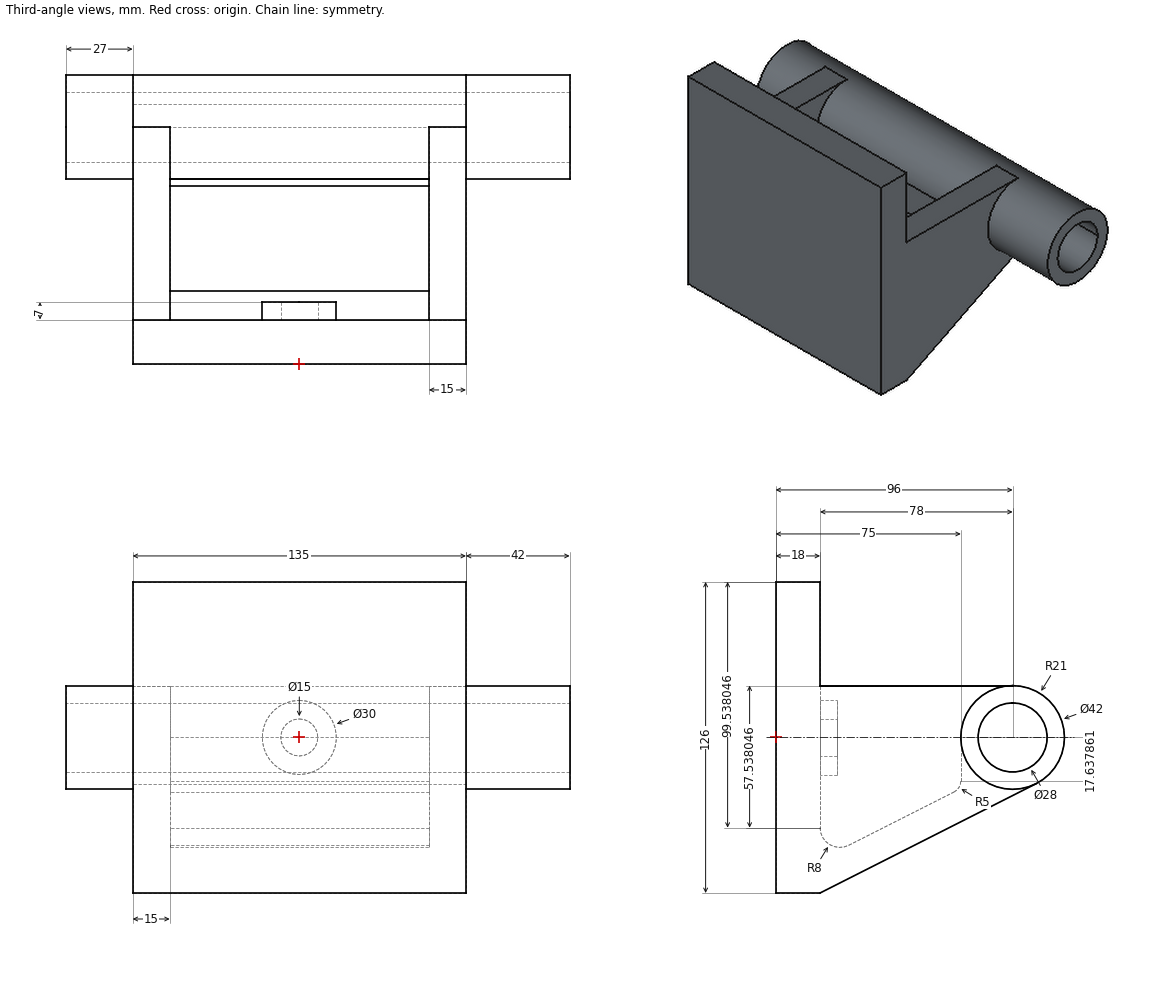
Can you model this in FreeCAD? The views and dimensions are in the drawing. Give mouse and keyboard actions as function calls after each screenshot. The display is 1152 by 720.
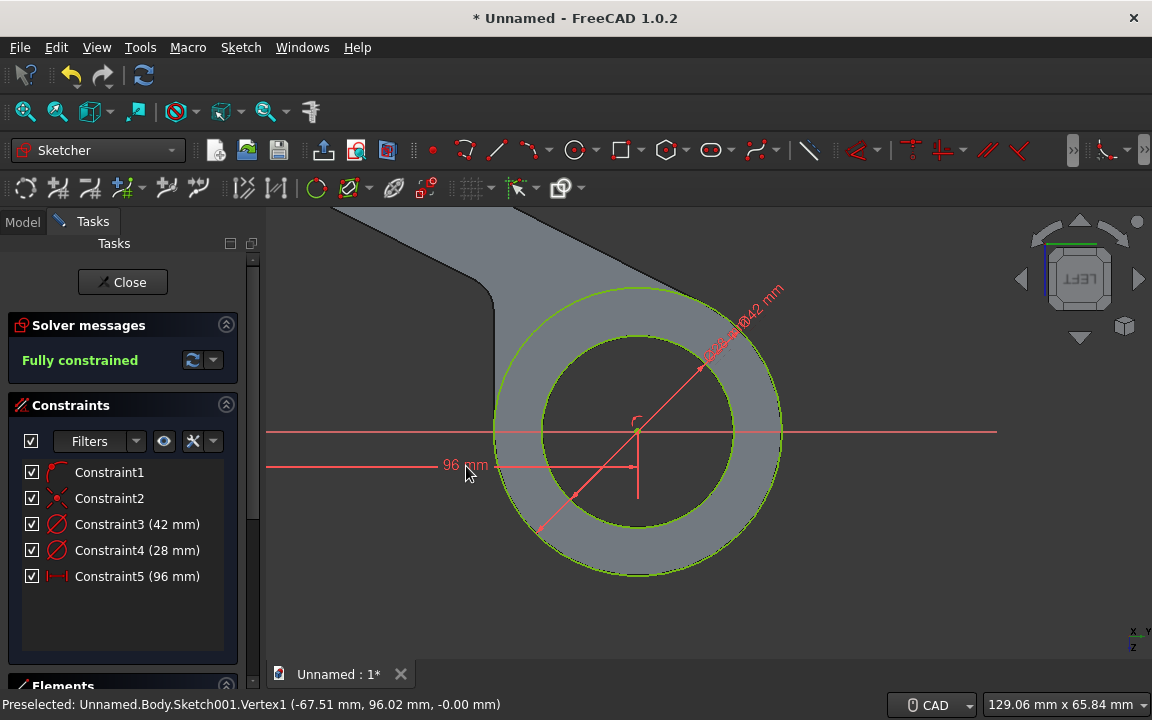
click(123, 282)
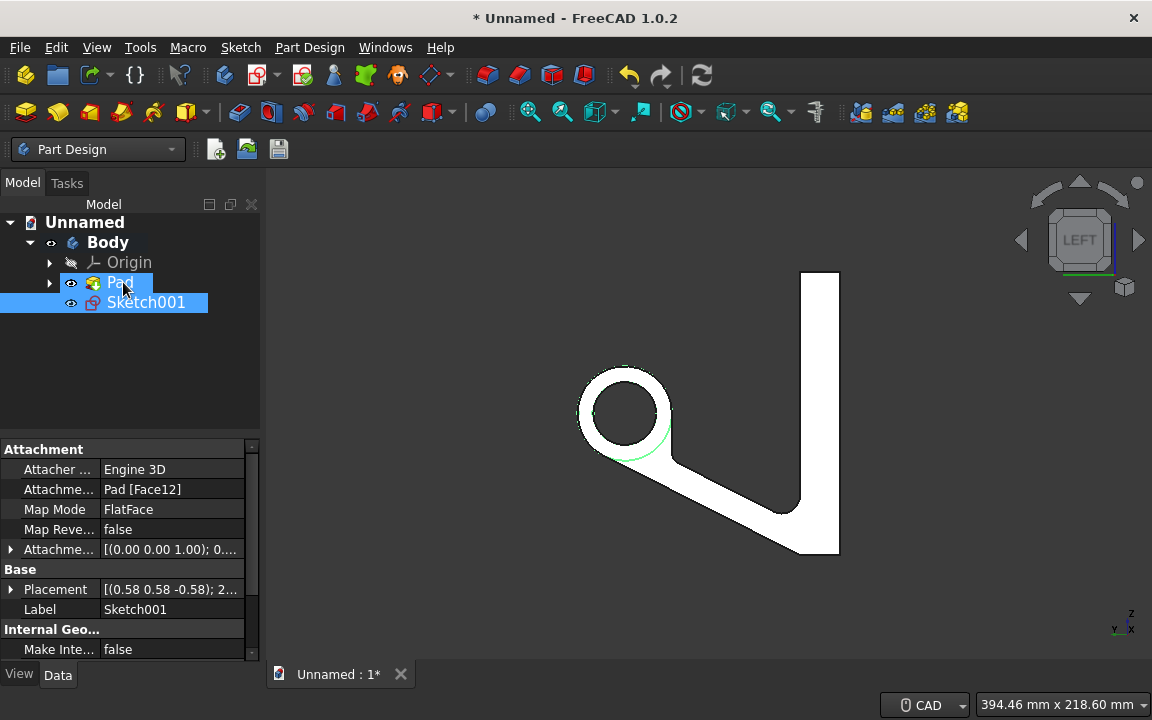
click(26, 112)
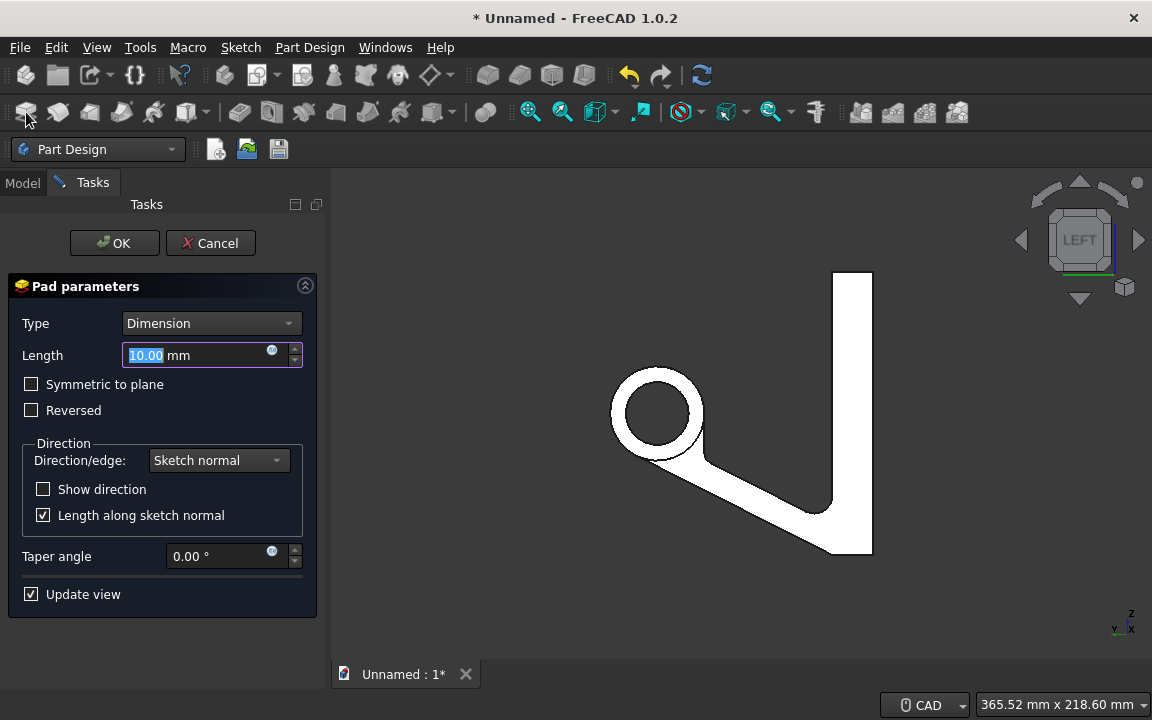
text(27)
key(Tab)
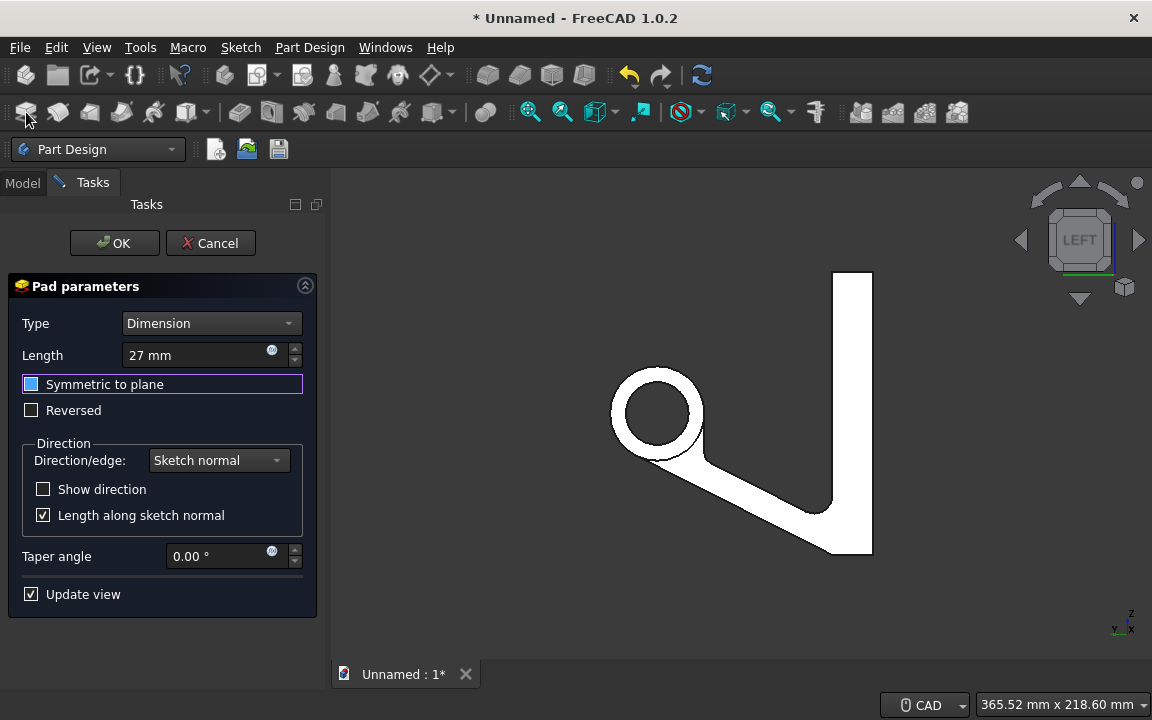
click(115, 243)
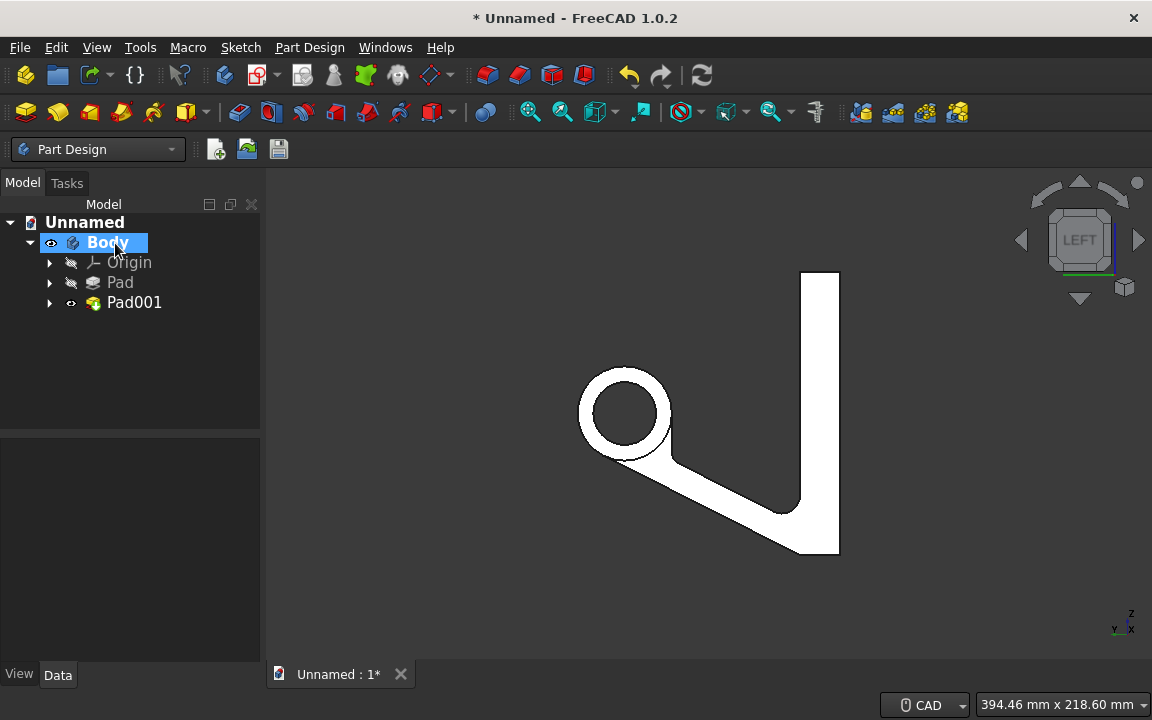
click(50, 263)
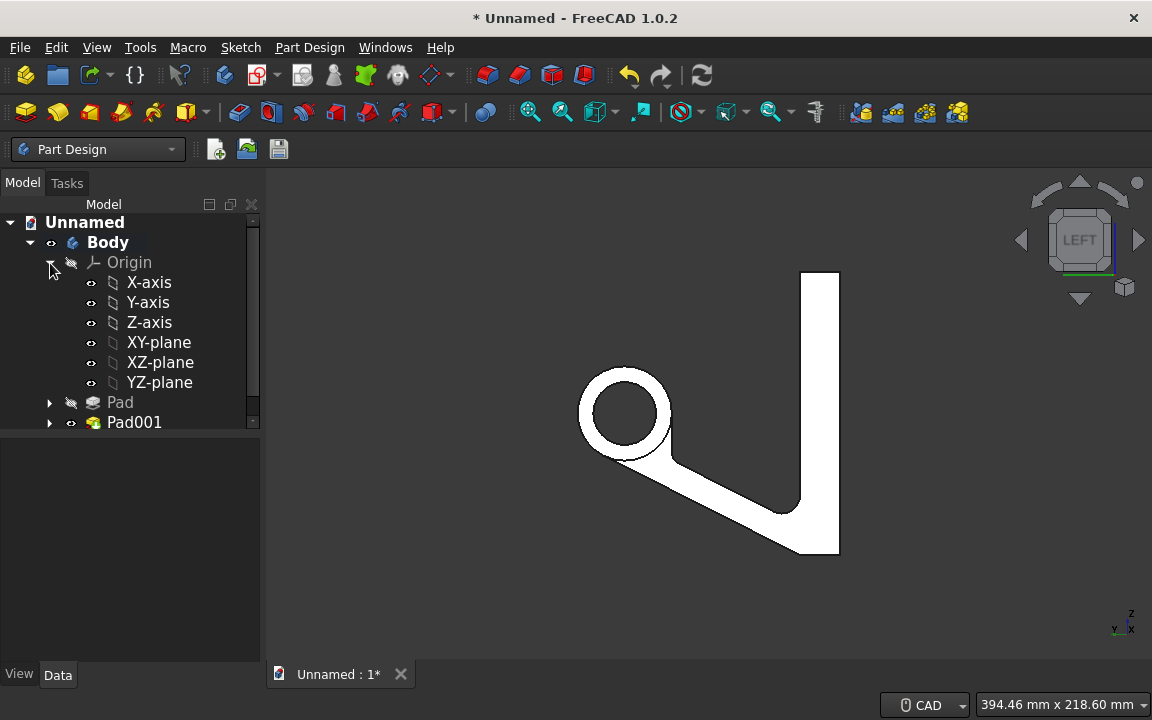
click(136, 383)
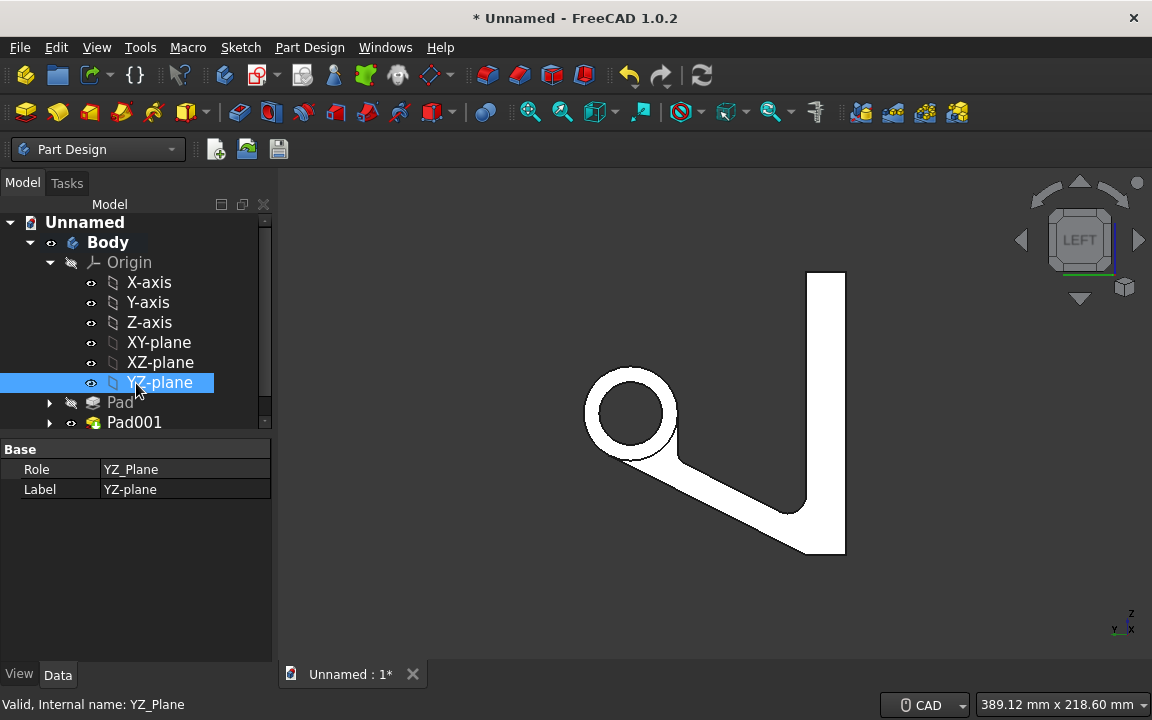
click(430, 76)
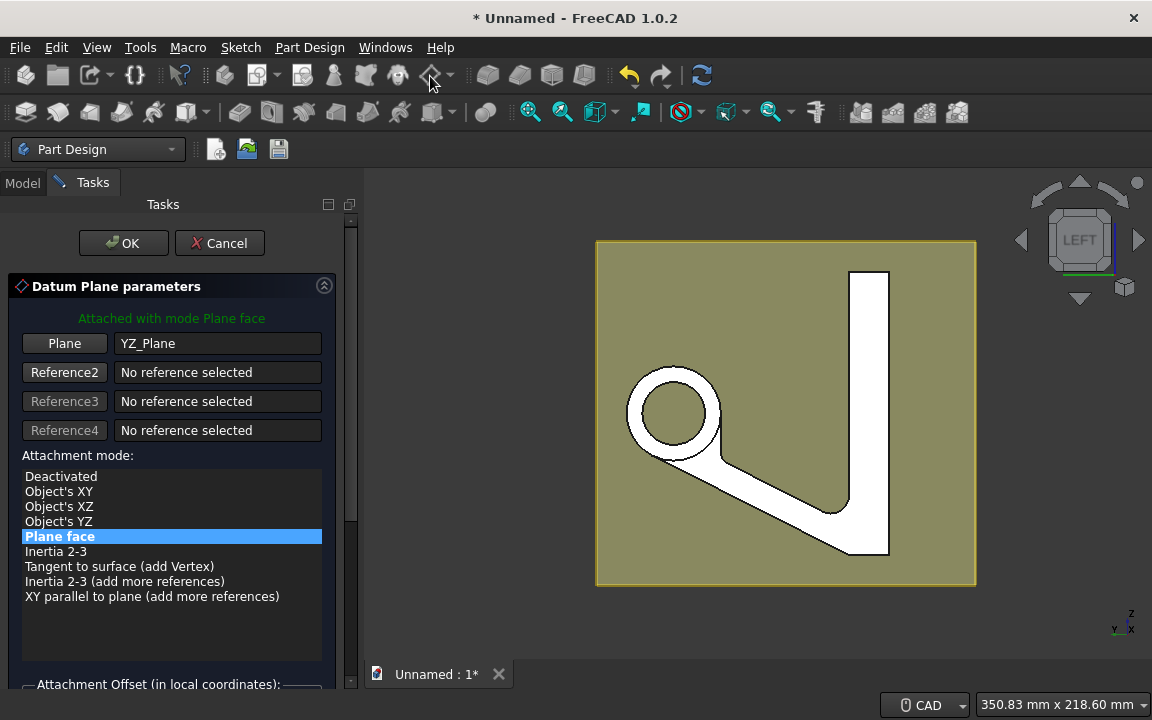
scroll(351, 451, down, 3)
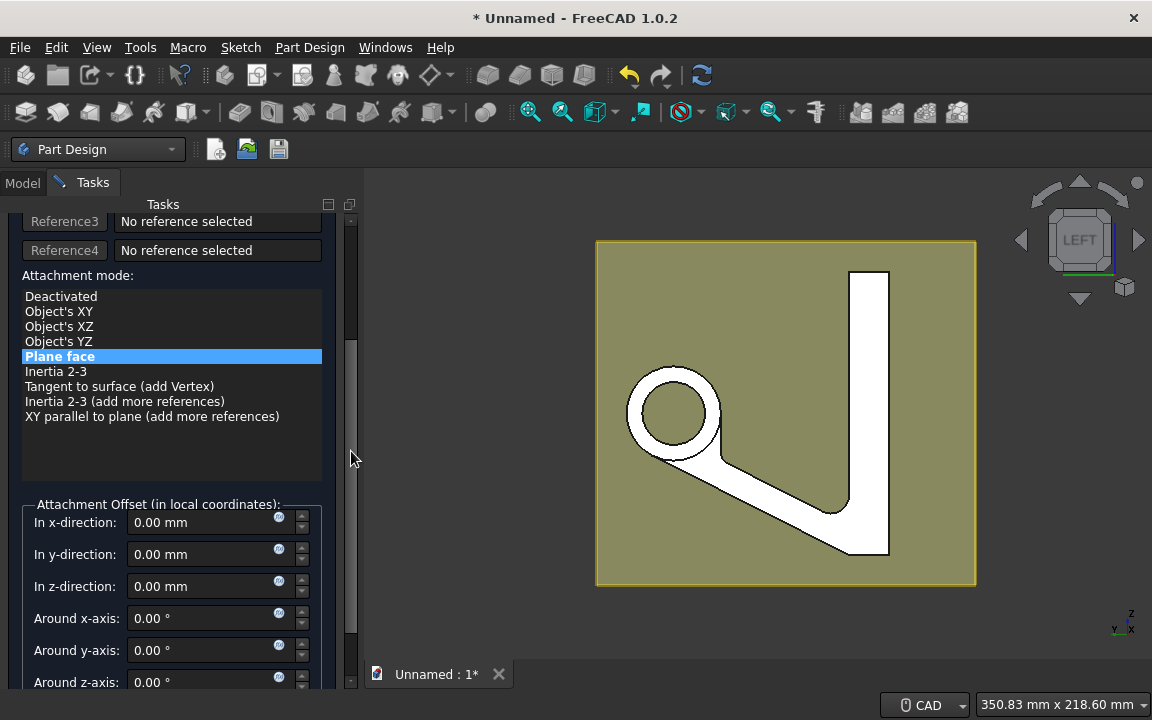
triple_click(210, 586)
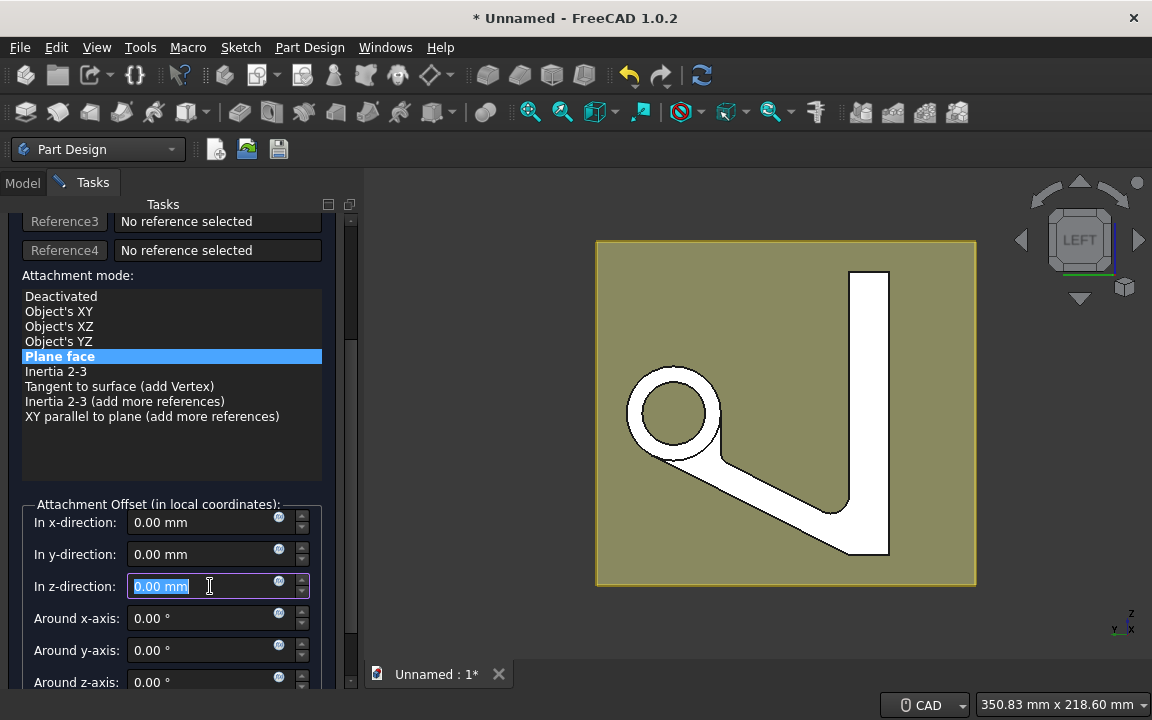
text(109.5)
key(Tab)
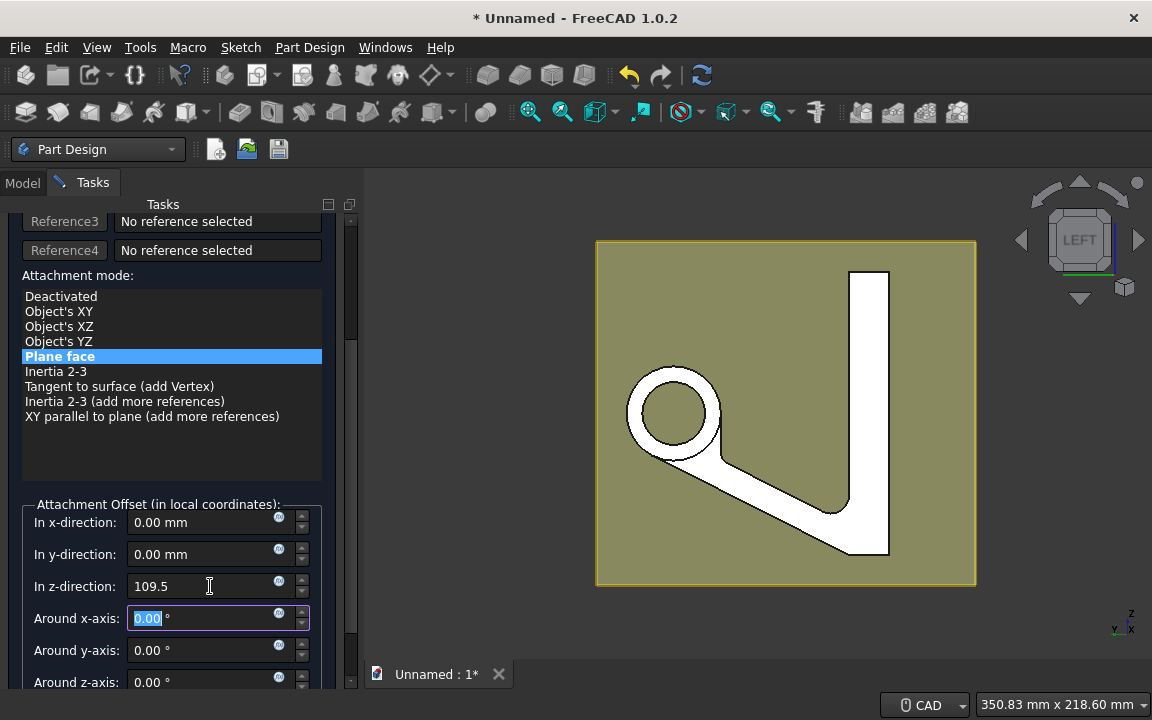
scroll(351, 451, up, 4)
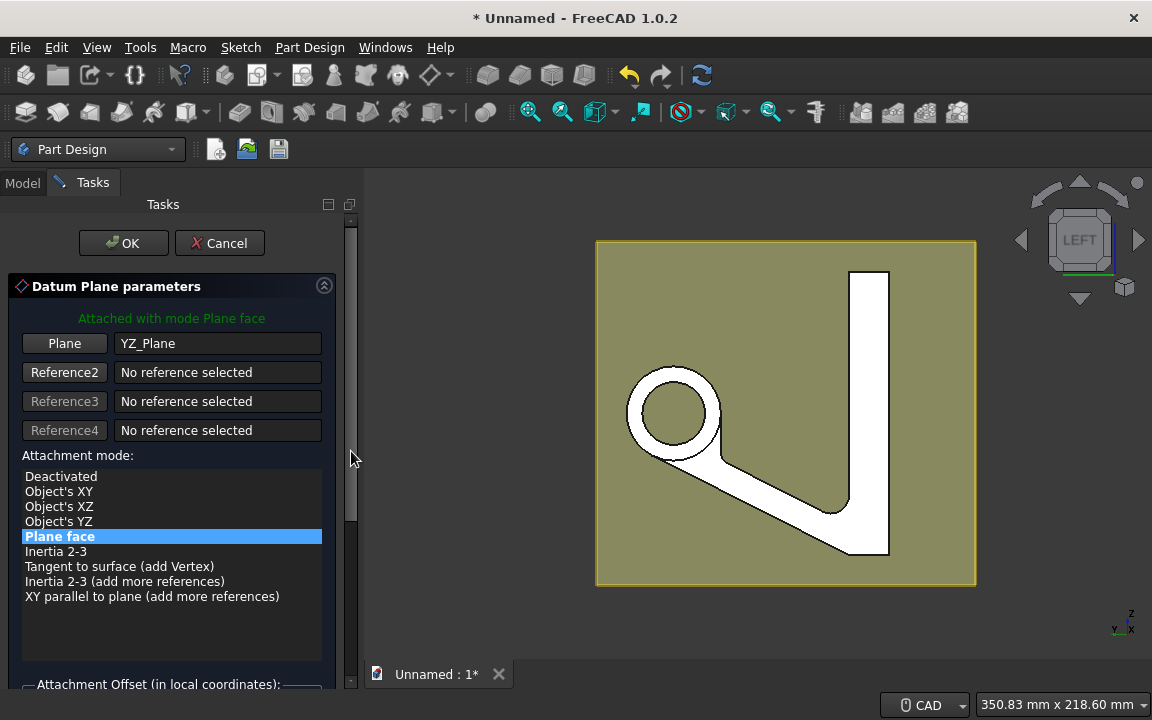
click(124, 243)